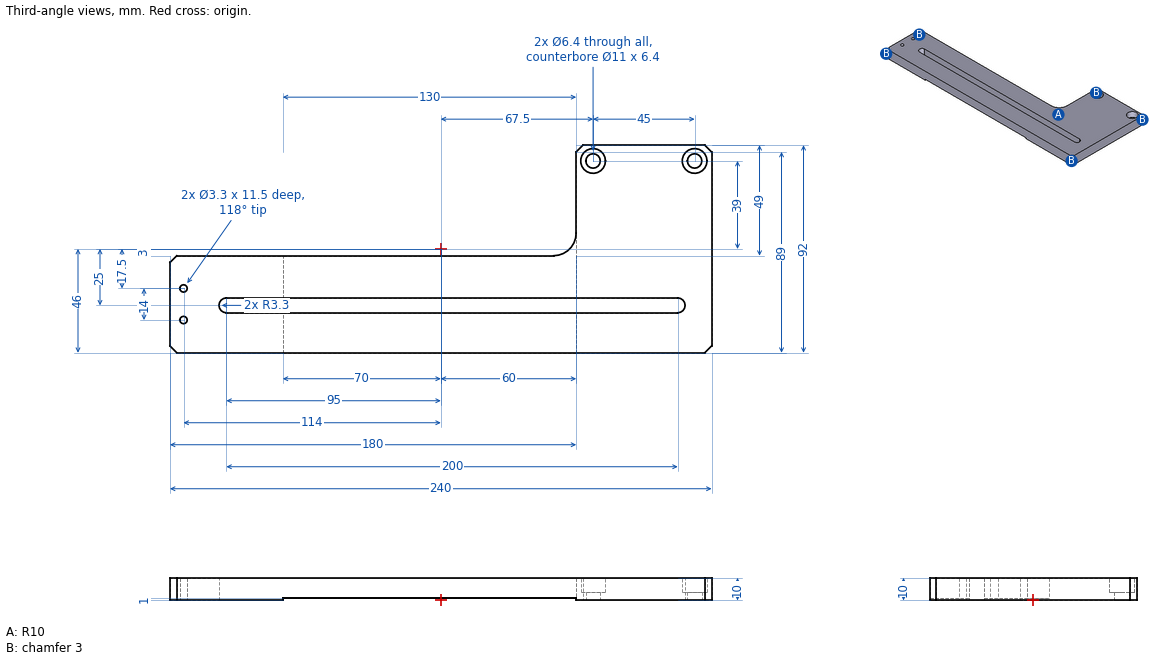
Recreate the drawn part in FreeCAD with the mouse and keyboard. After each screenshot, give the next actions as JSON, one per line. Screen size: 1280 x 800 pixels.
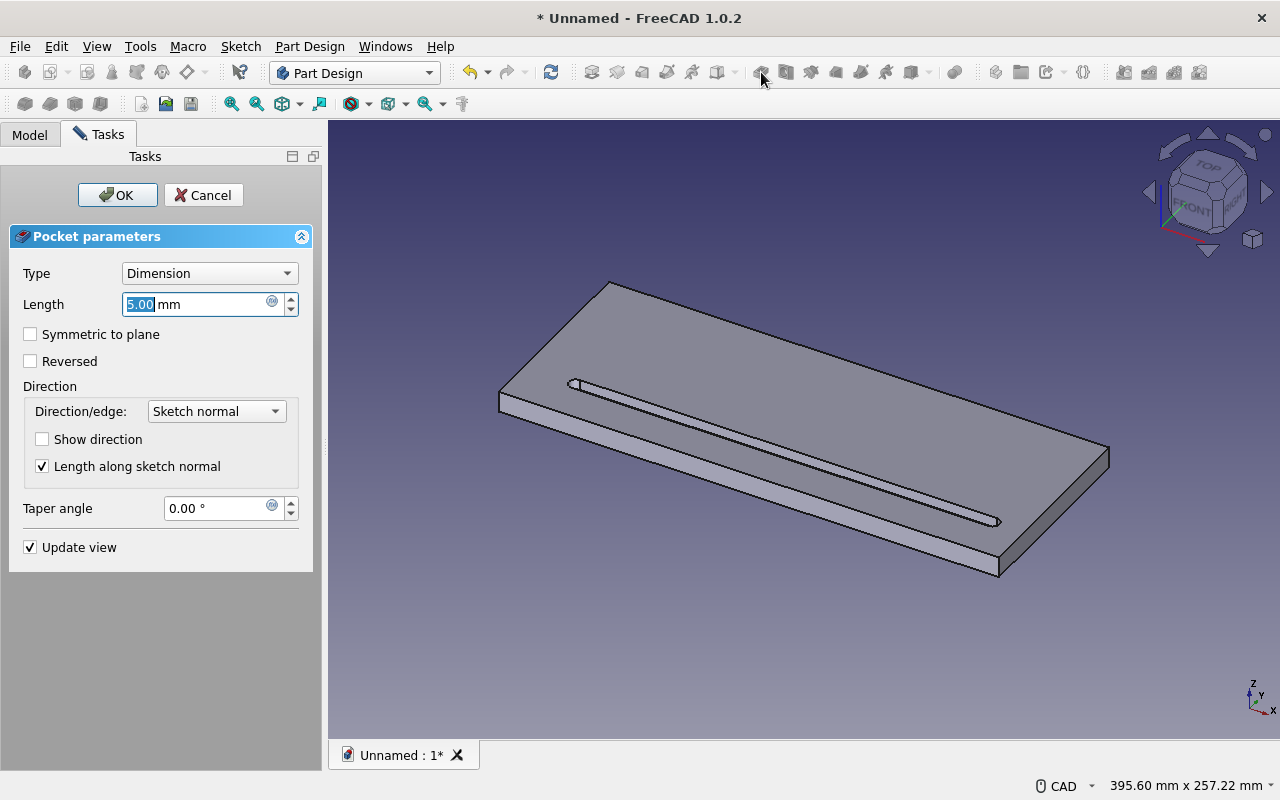
{"action": "type", "text": "10"}
{"action": "key", "text": "Tab"}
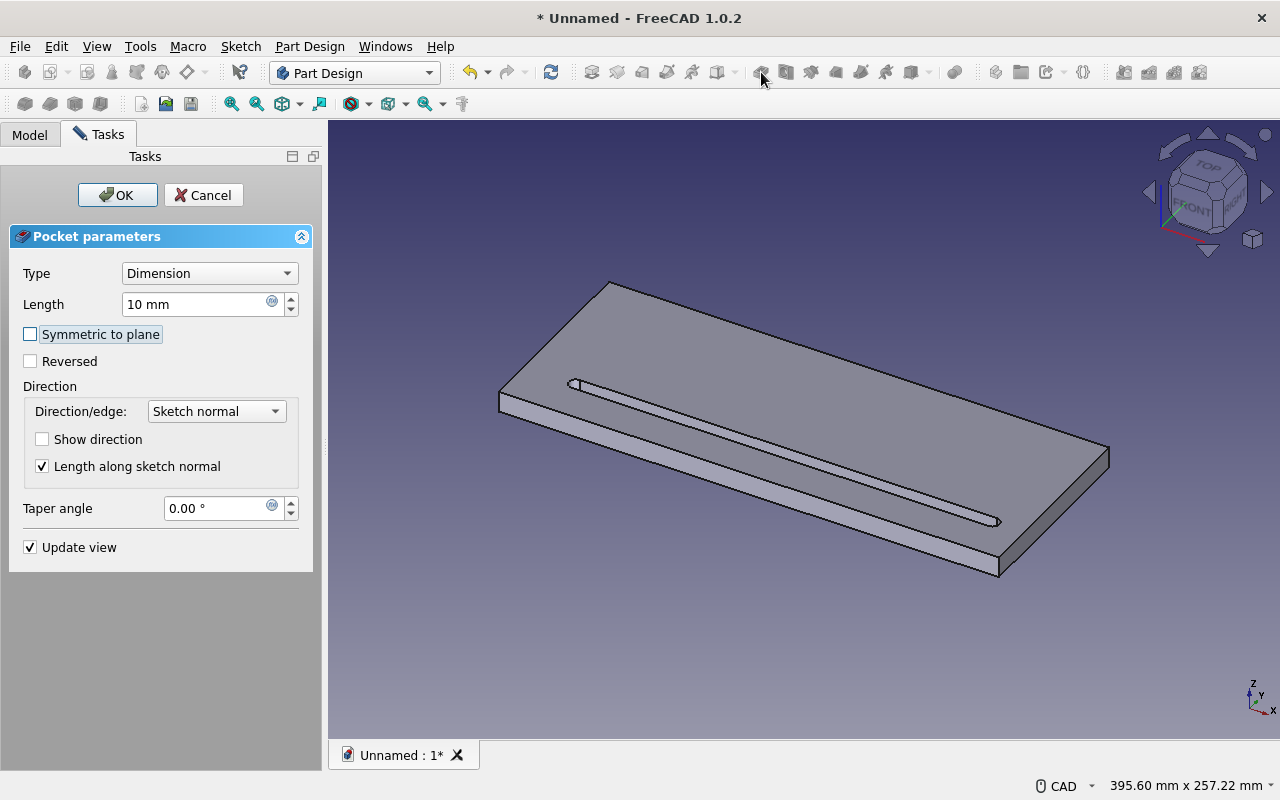
{"action": "left_click", "coordinate": [118, 195]}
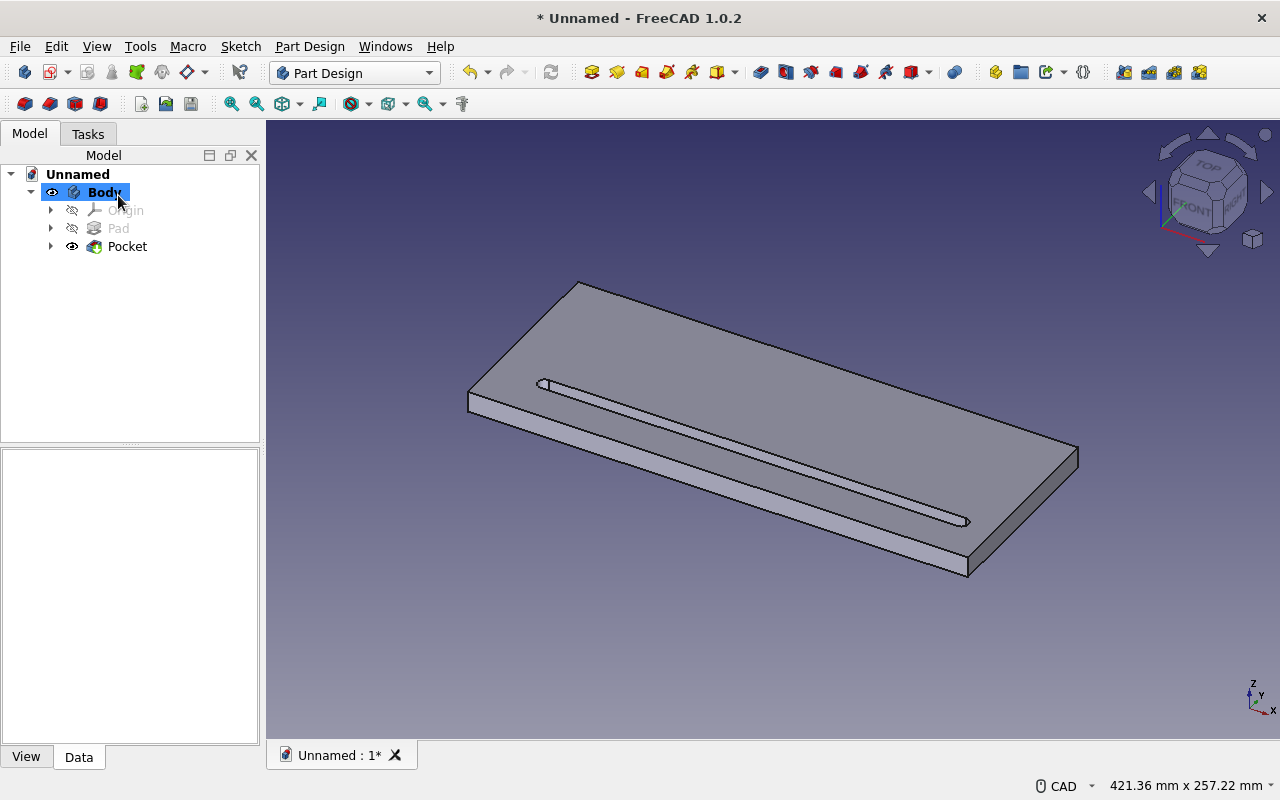
{"action": "left_click", "coordinate": [932, 450]}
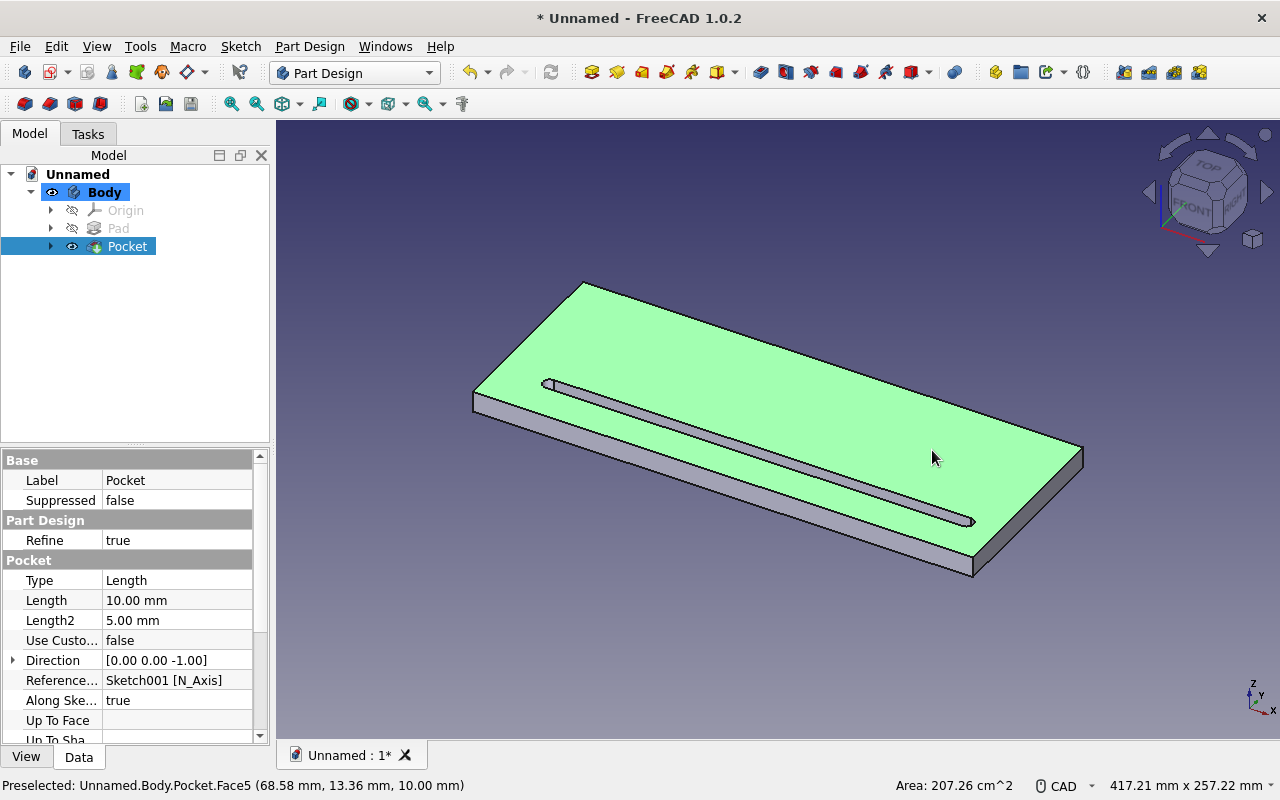
{"action": "left_click", "coordinate": [50, 72]}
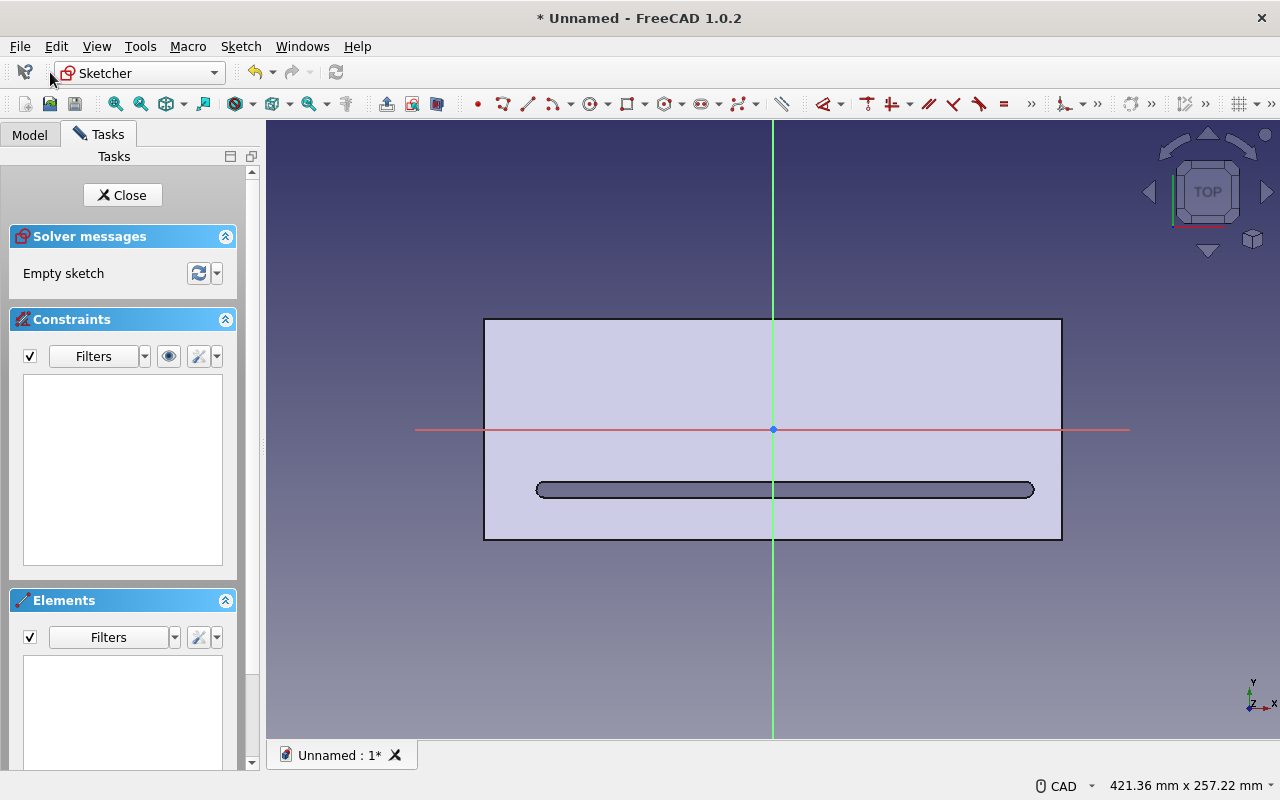
{"action": "left_click", "coordinate": [626, 104]}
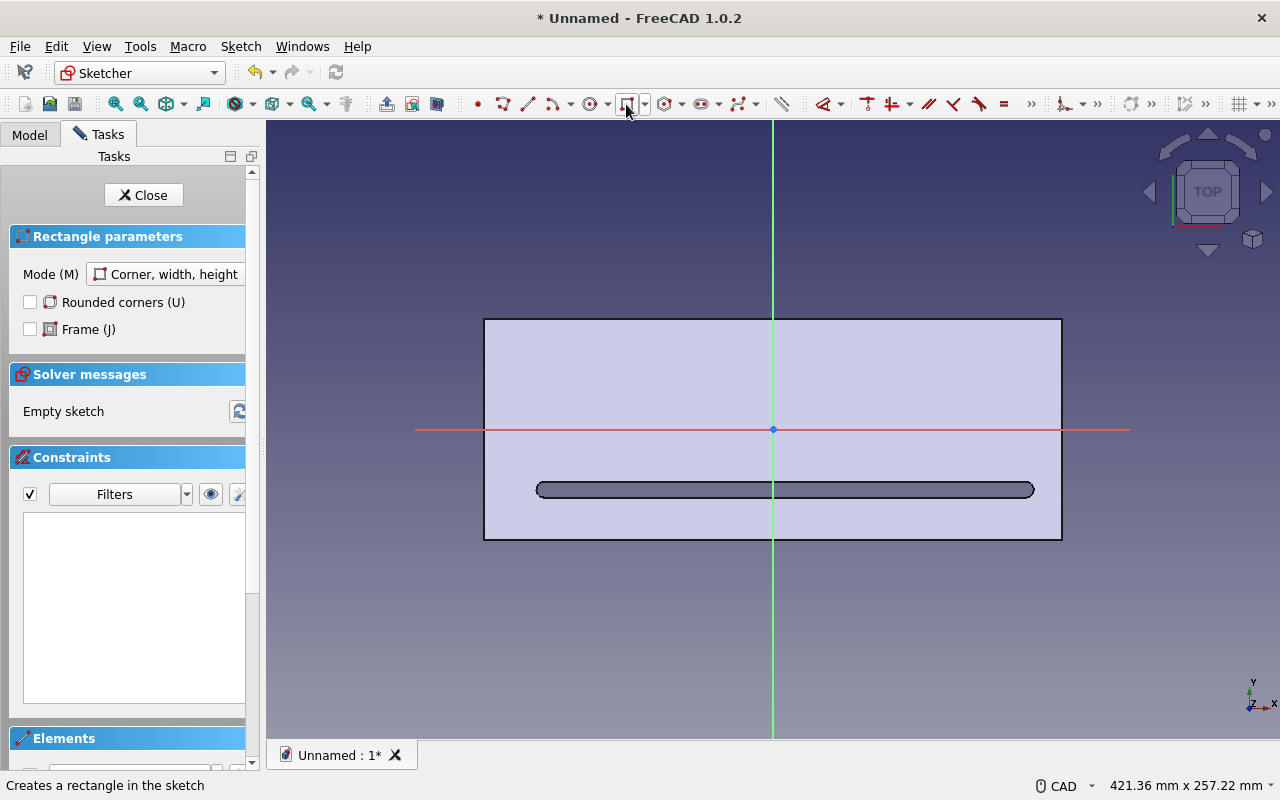
{"action": "left_click", "coordinate": [484, 319]}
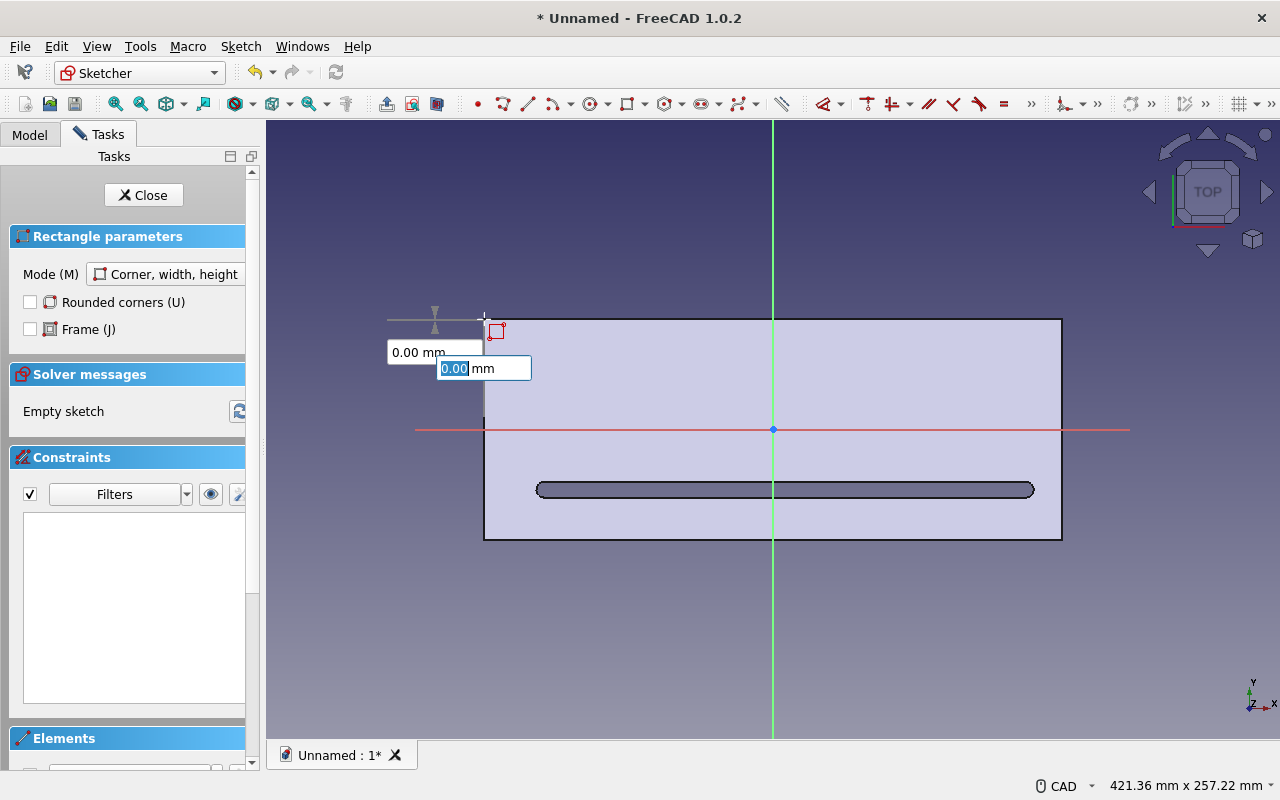
{"action": "scroll", "coordinate": [917, 437], "scroll_direction": "up", "scroll_amount": 4}
{"action": "mouse_move", "coordinate": [917, 436]}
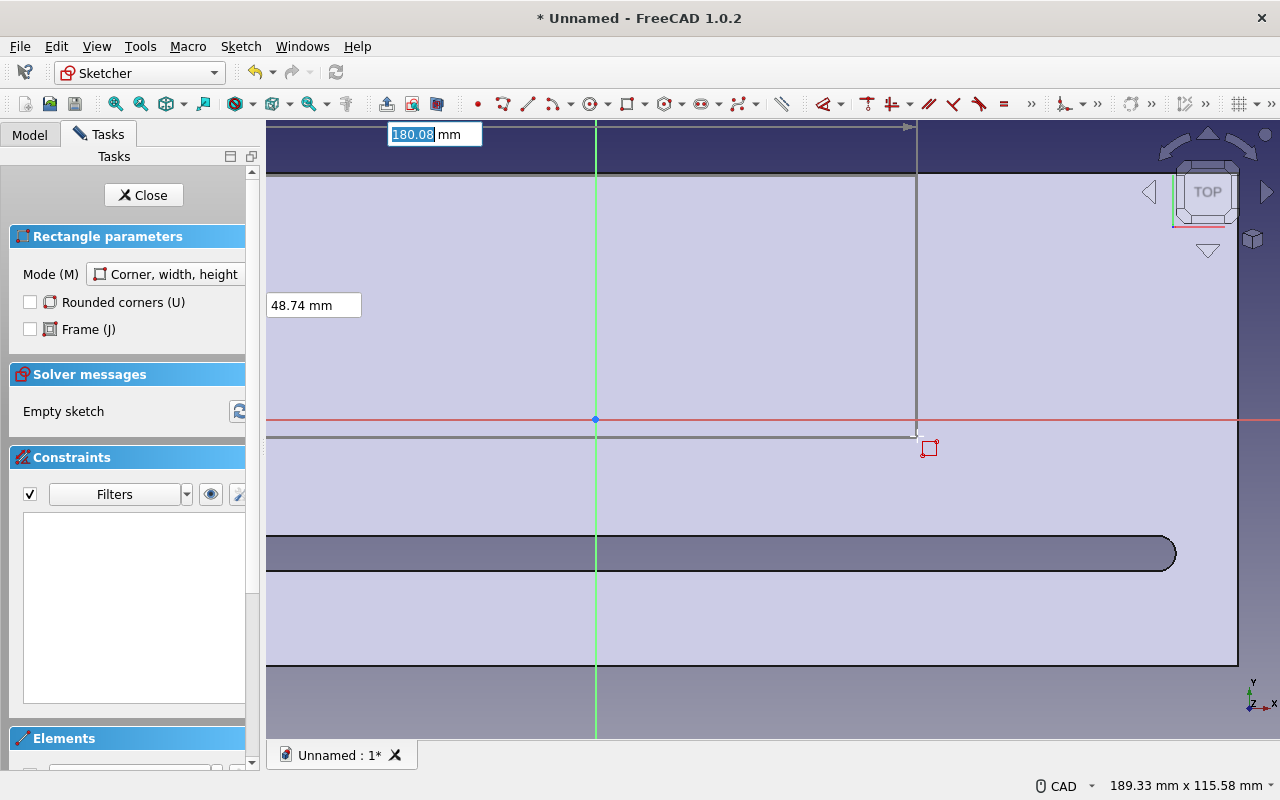
{"action": "type", "text": "180"}
{"action": "key", "text": "Tab"}
{"action": "type", "text": "49"}
{"action": "key", "text": "Return"}
{"action": "key", "text": "Escape"}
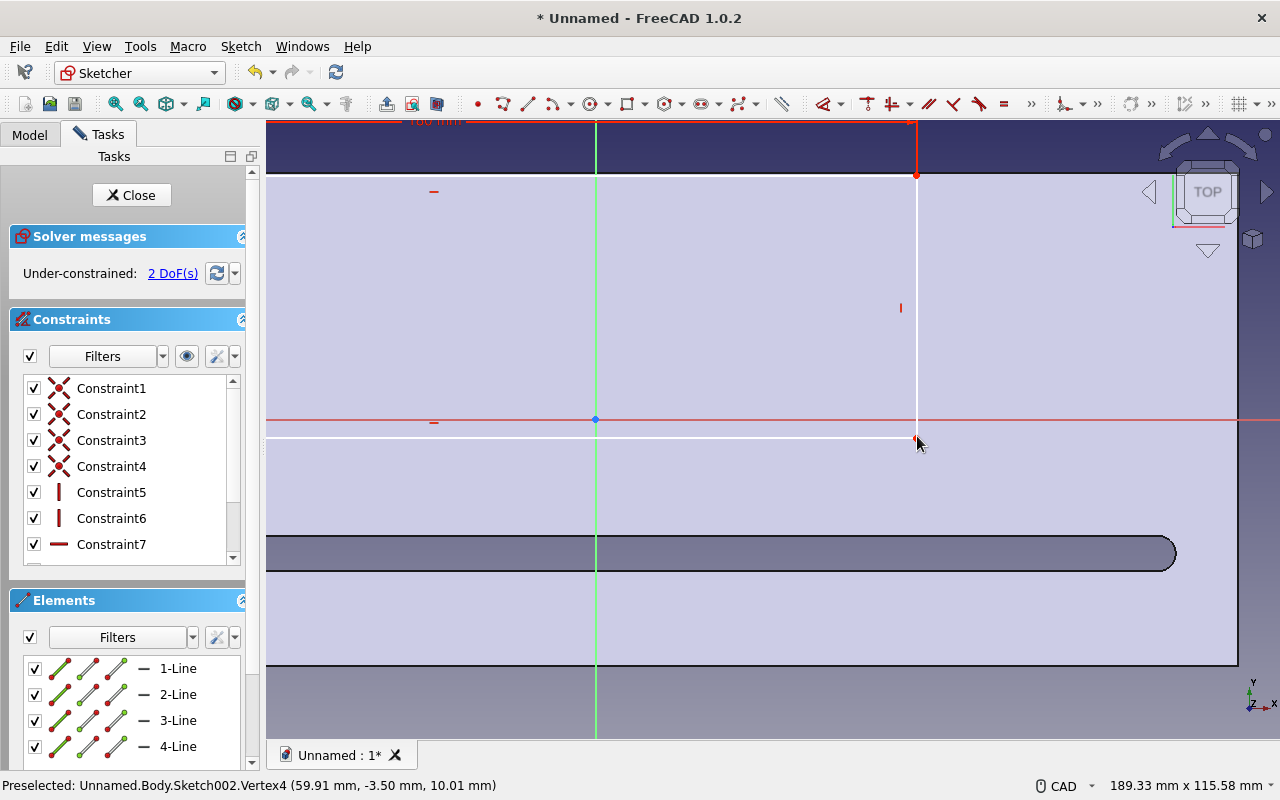
{"action": "scroll", "coordinate": [1032, 582], "scroll_direction": "down", "scroll_amount": 3}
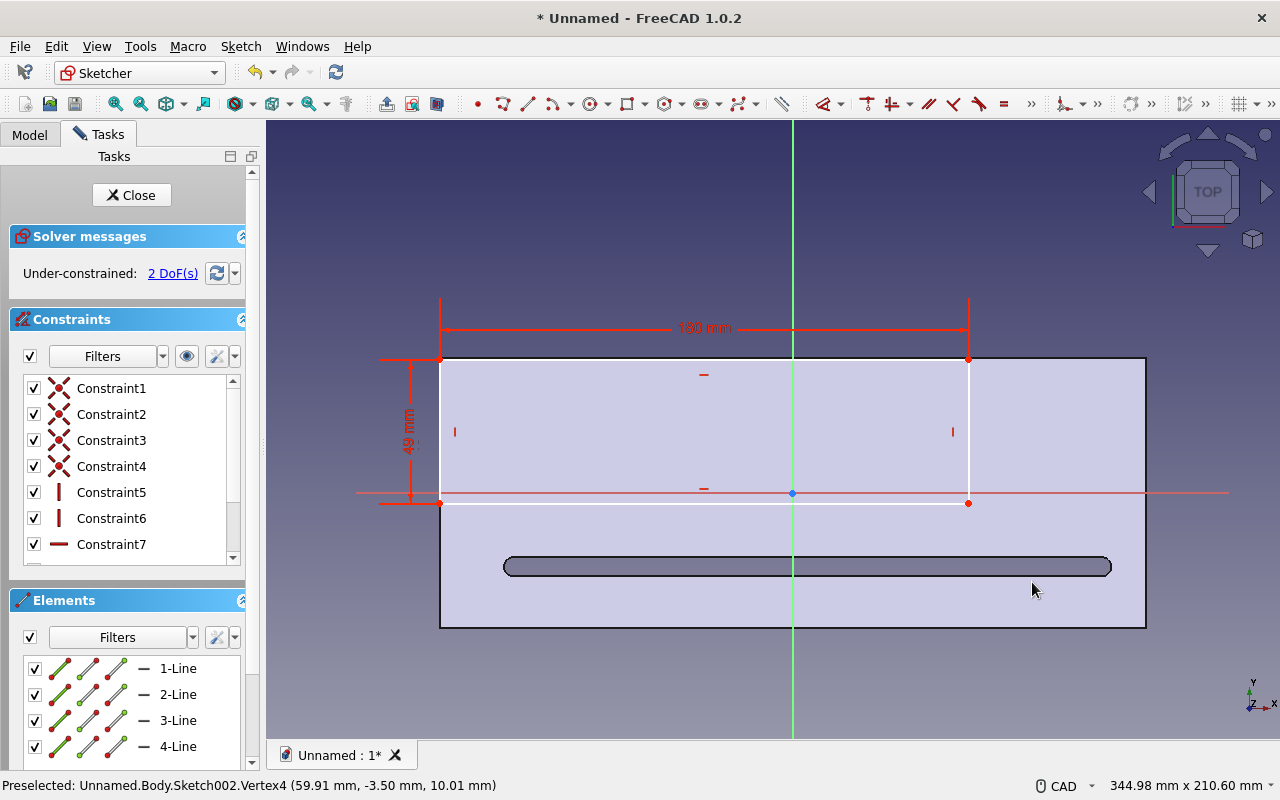
{"action": "scroll", "coordinate": [440, 504], "scroll_direction": "up", "scroll_amount": 8}